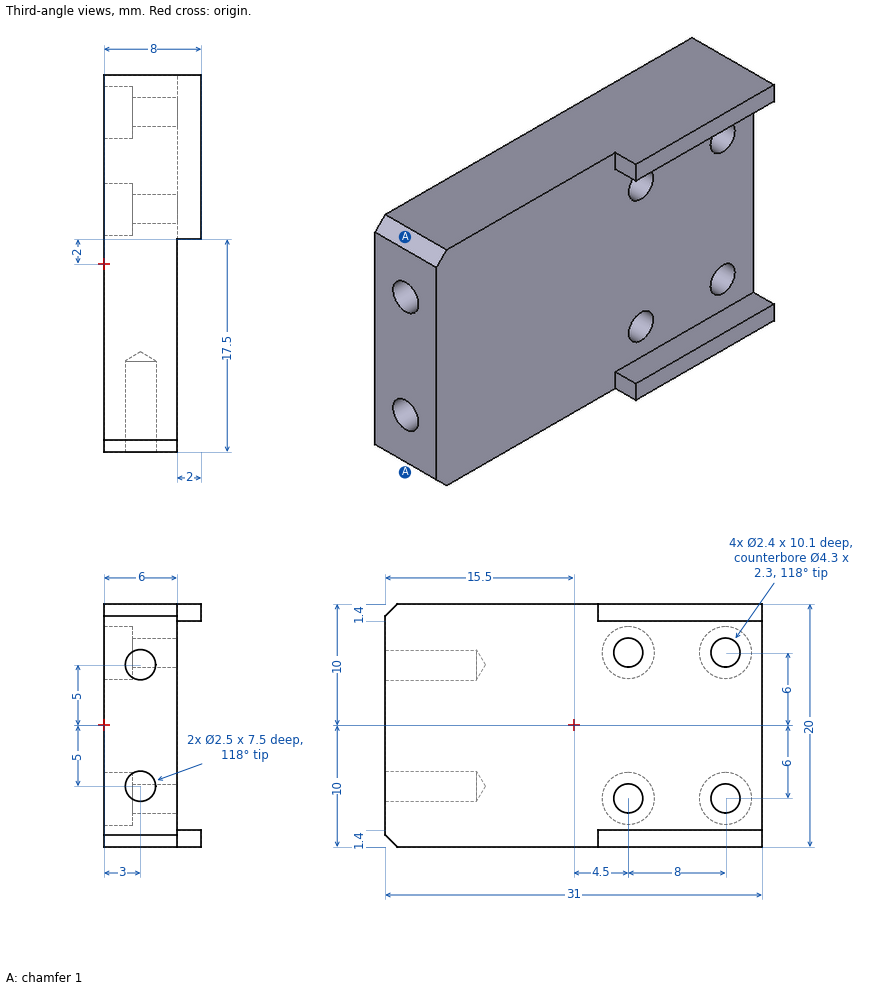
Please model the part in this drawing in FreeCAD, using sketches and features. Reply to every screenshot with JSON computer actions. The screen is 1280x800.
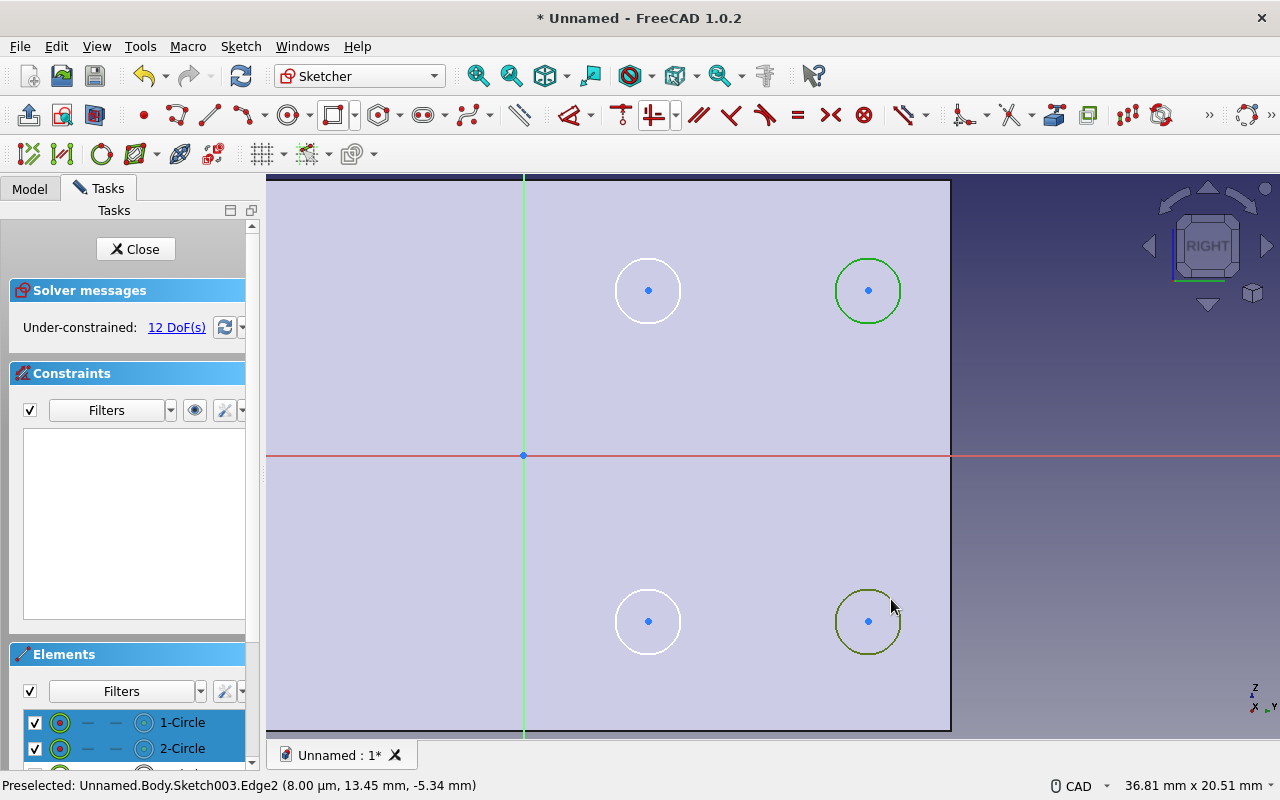
{"action": "left_click", "coordinate": [671, 599]}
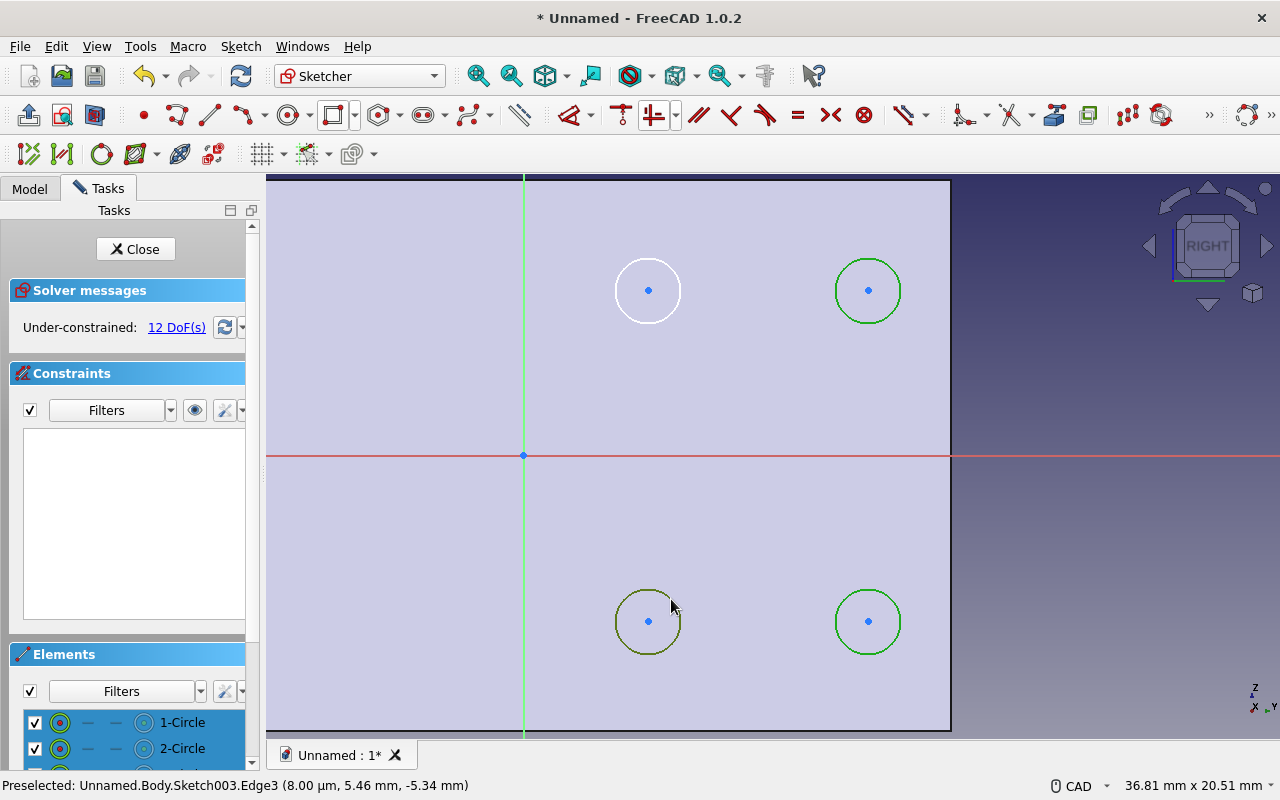
{"action": "left_click", "coordinate": [671, 268]}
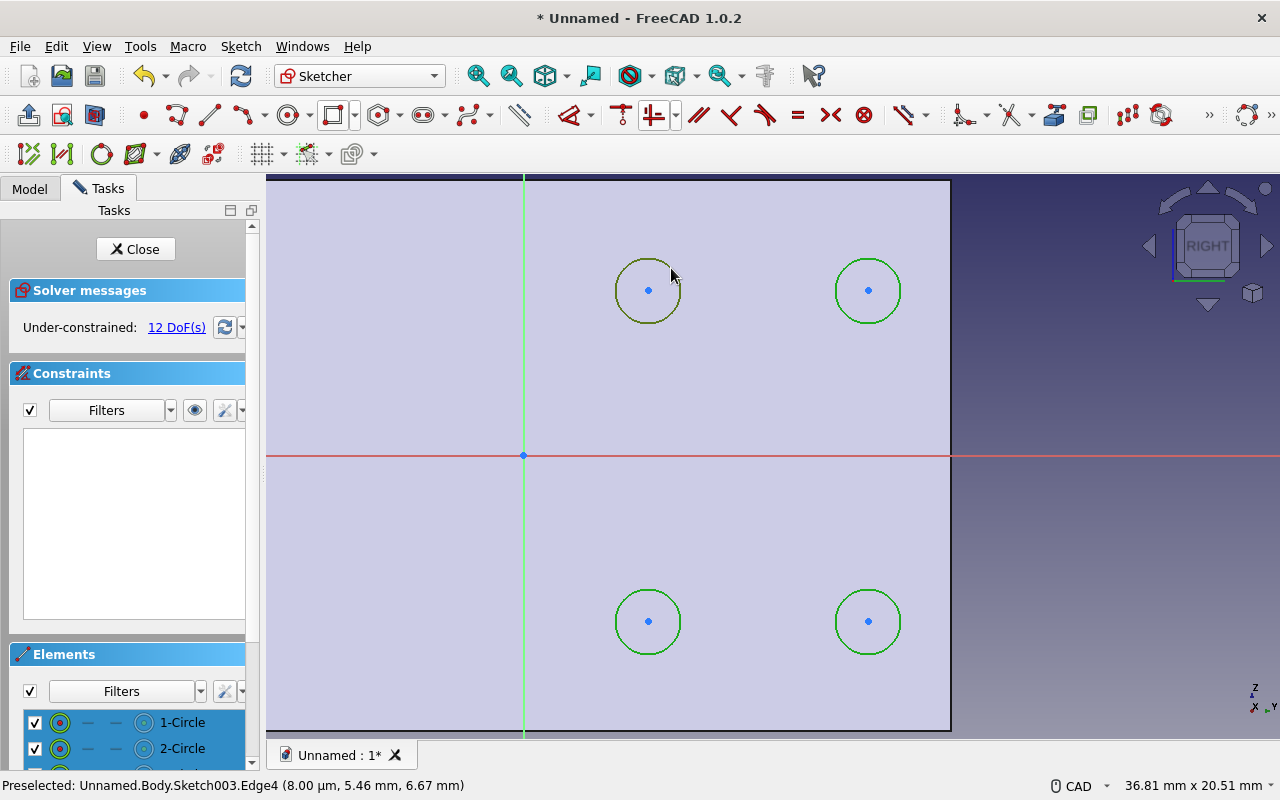
{"action": "left_click", "coordinate": [798, 116]}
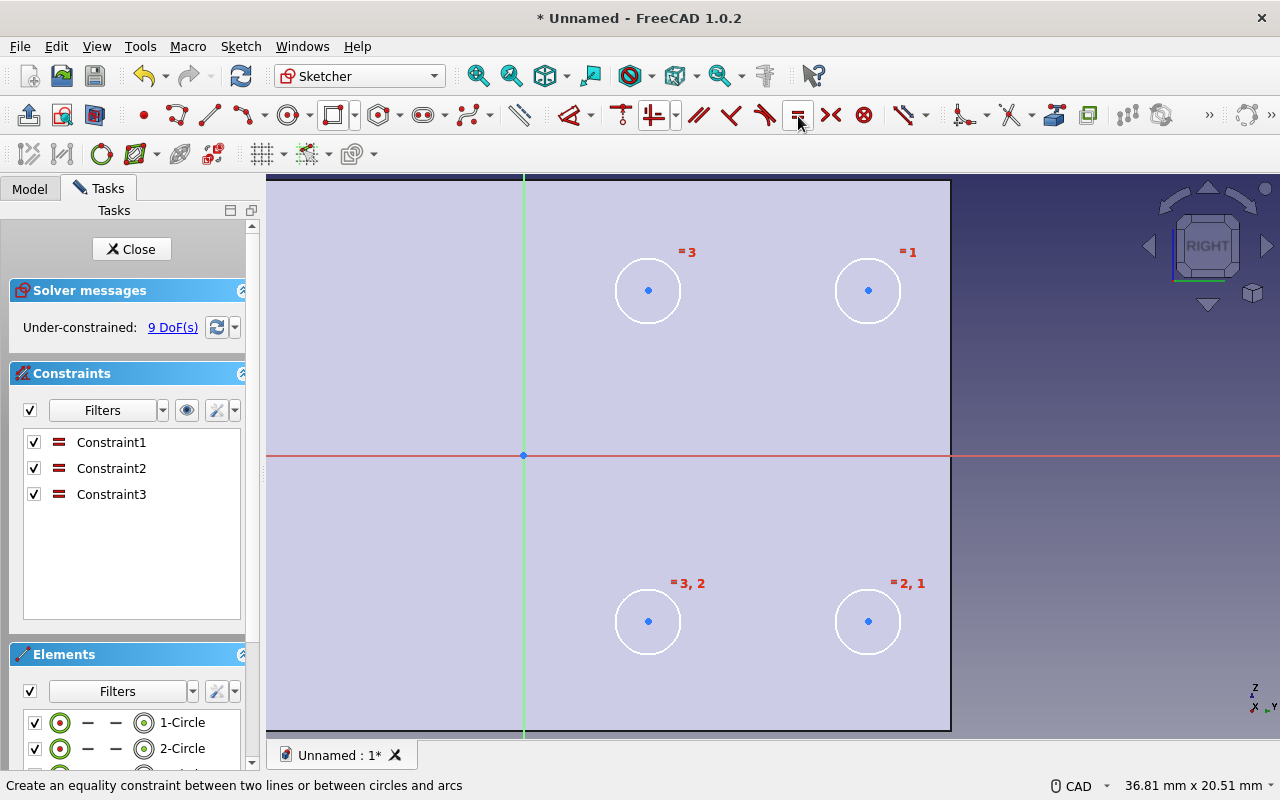
{"action": "left_click", "coordinate": [868, 291]}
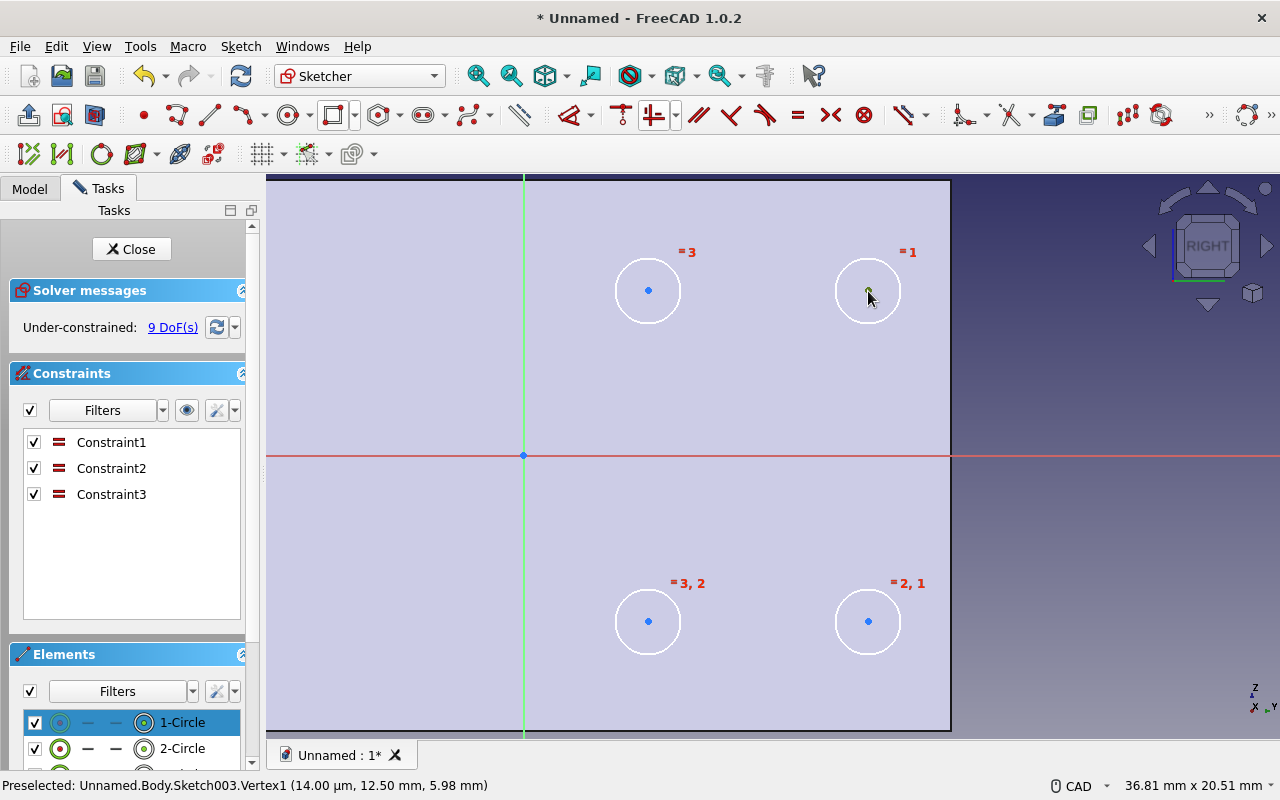
{"action": "left_click", "coordinate": [868, 622]}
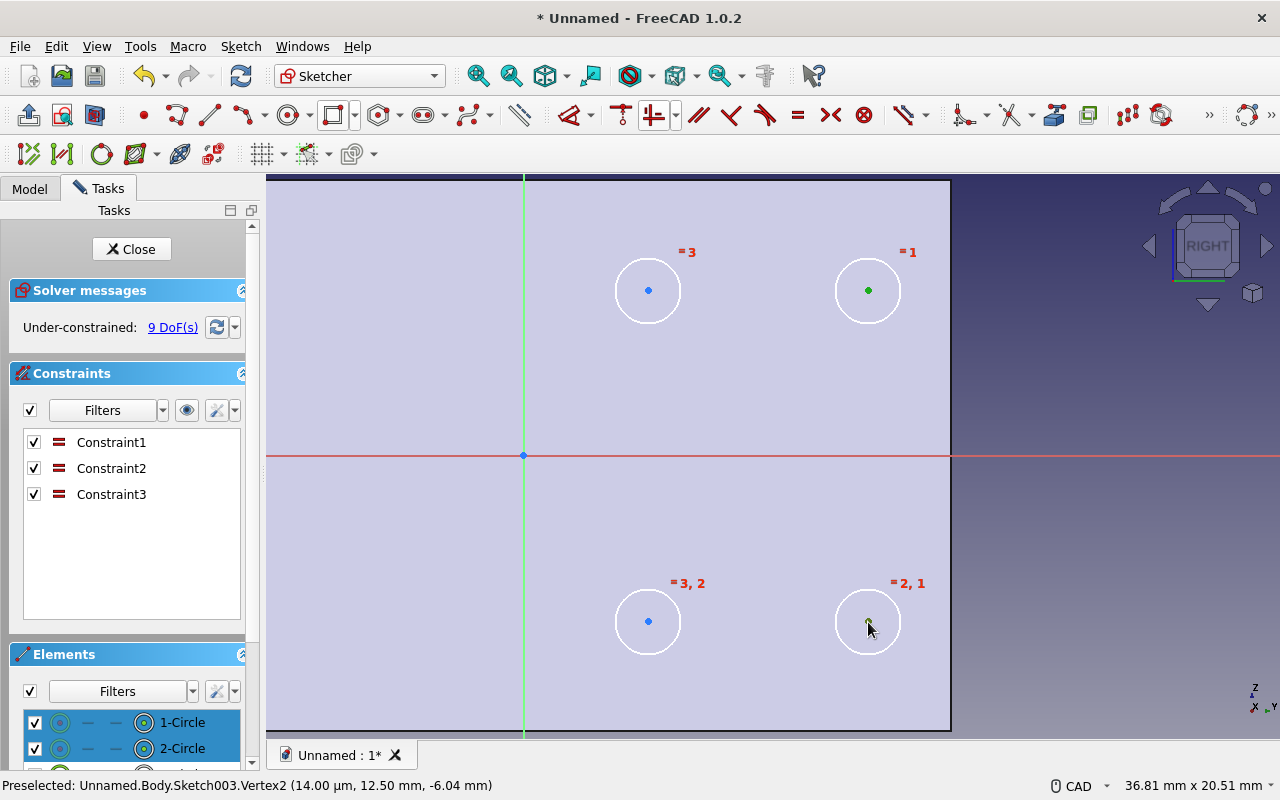
{"action": "left_click", "coordinate": [676, 116]}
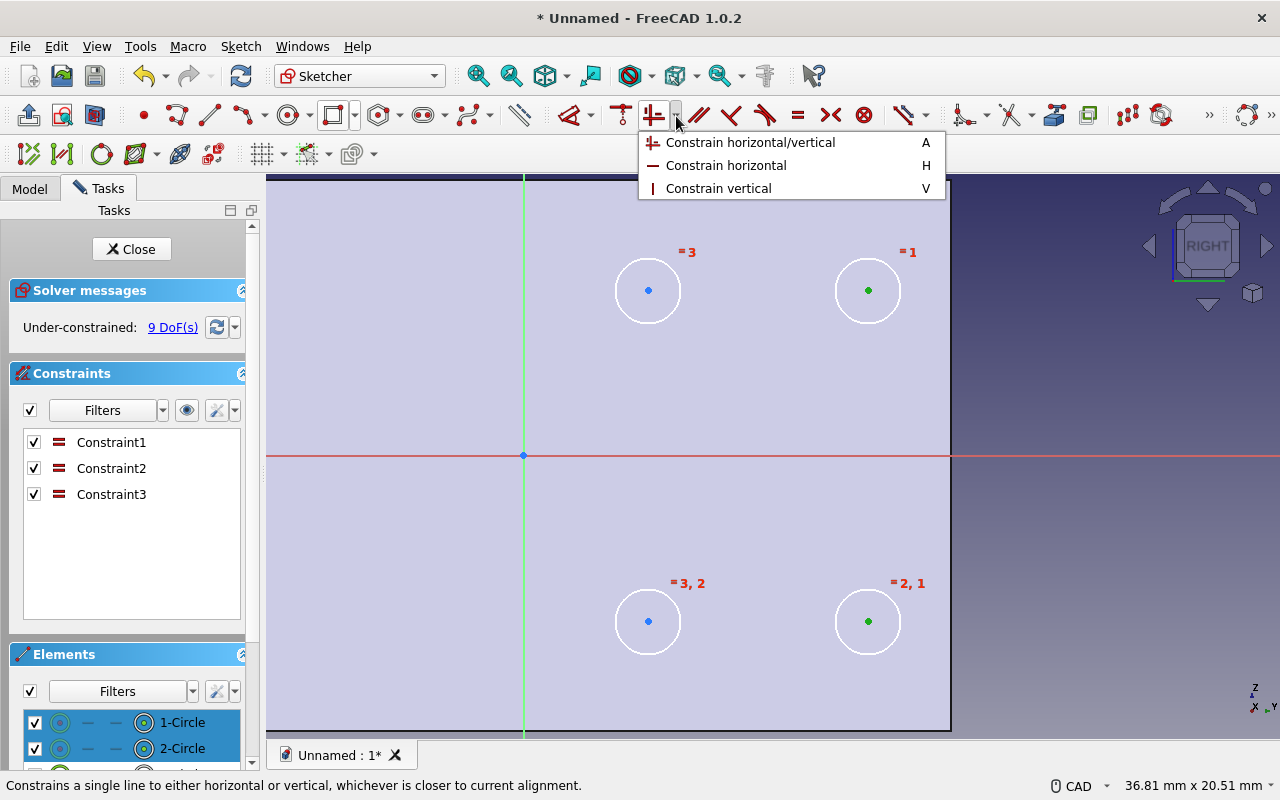
{"action": "left_click", "coordinate": [792, 188]}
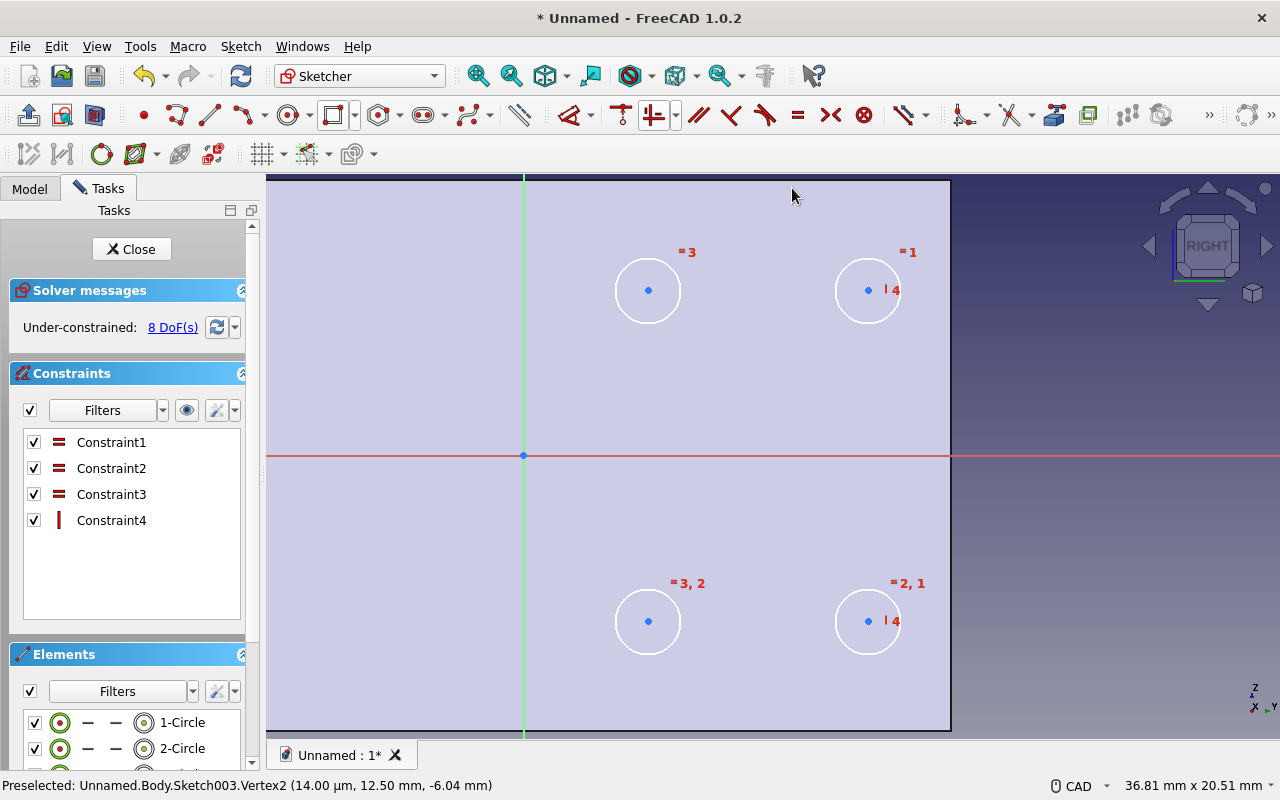
{"action": "left_click", "coordinate": [868, 622]}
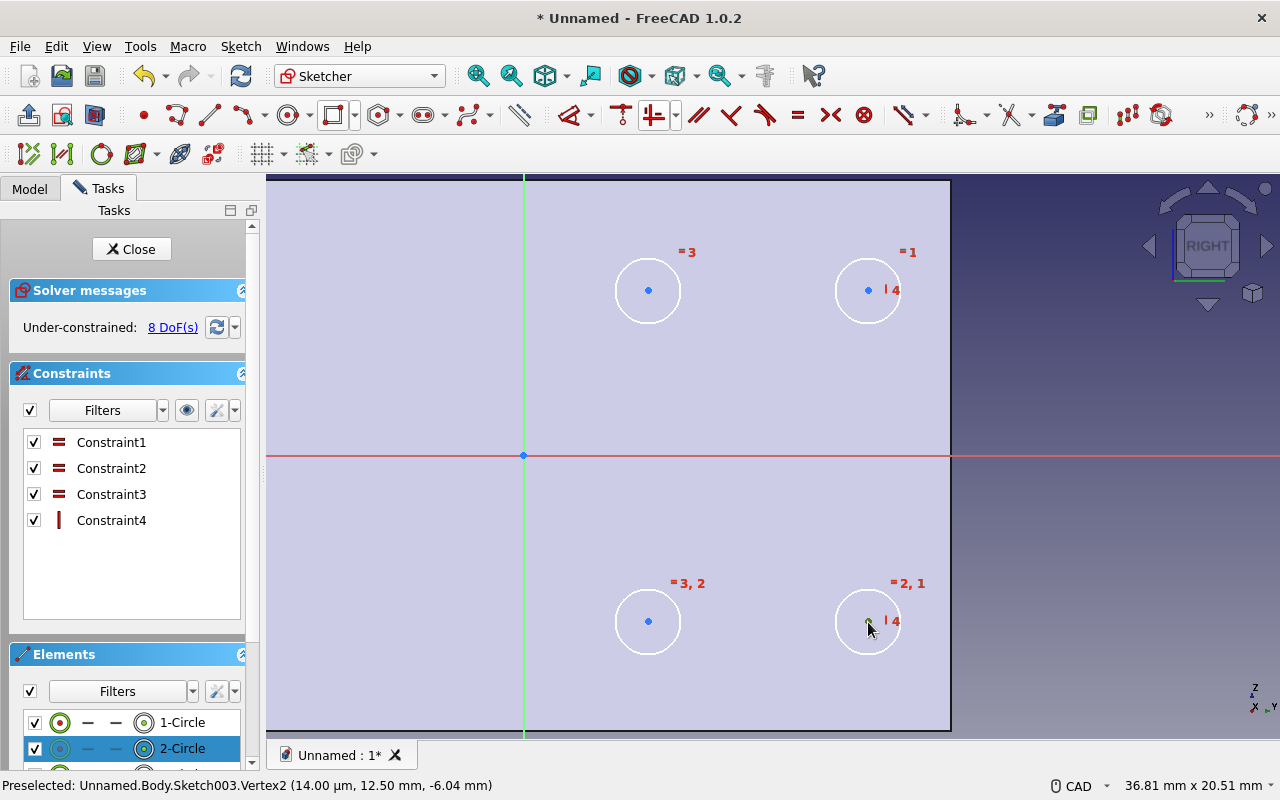
{"action": "left_click", "coordinate": [648, 622]}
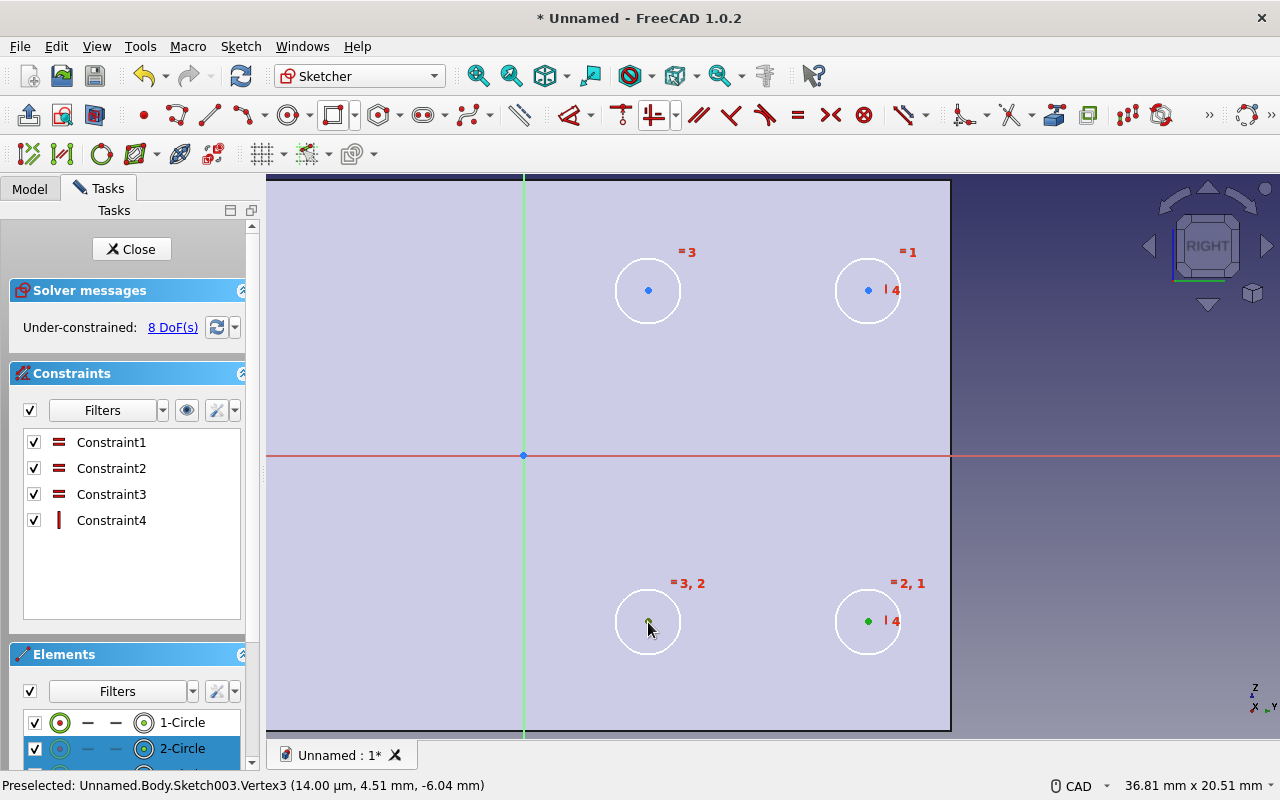
{"action": "key", "text": "h"}